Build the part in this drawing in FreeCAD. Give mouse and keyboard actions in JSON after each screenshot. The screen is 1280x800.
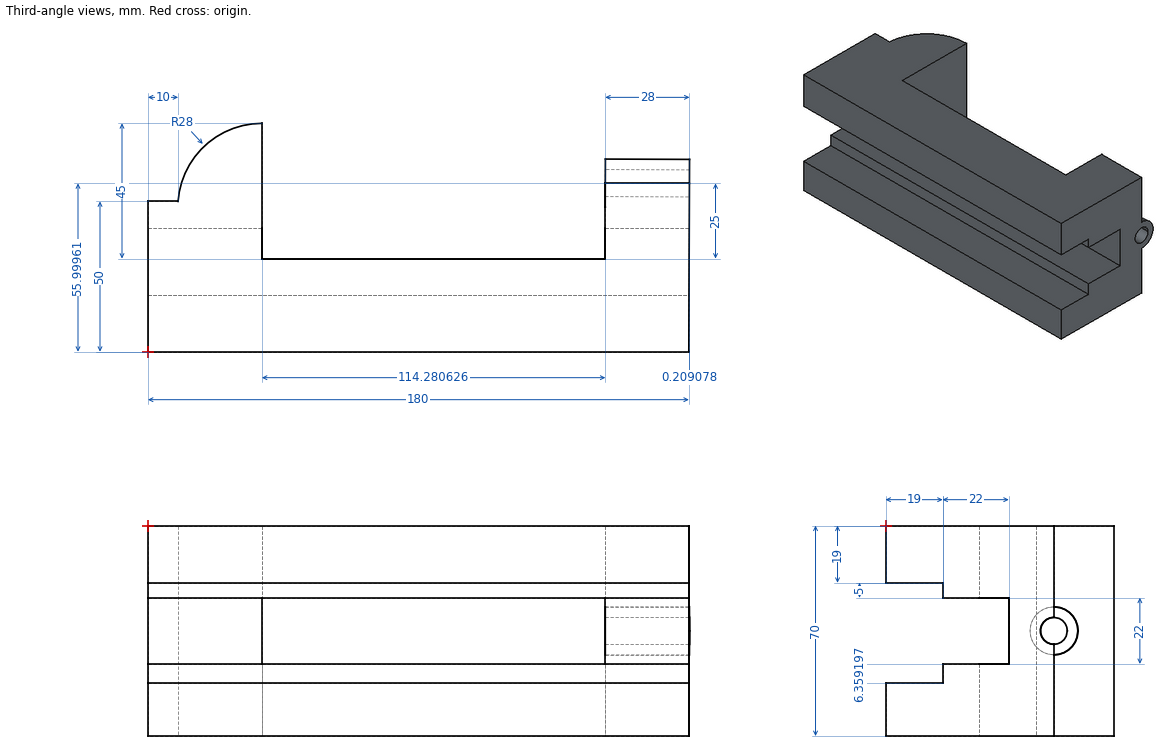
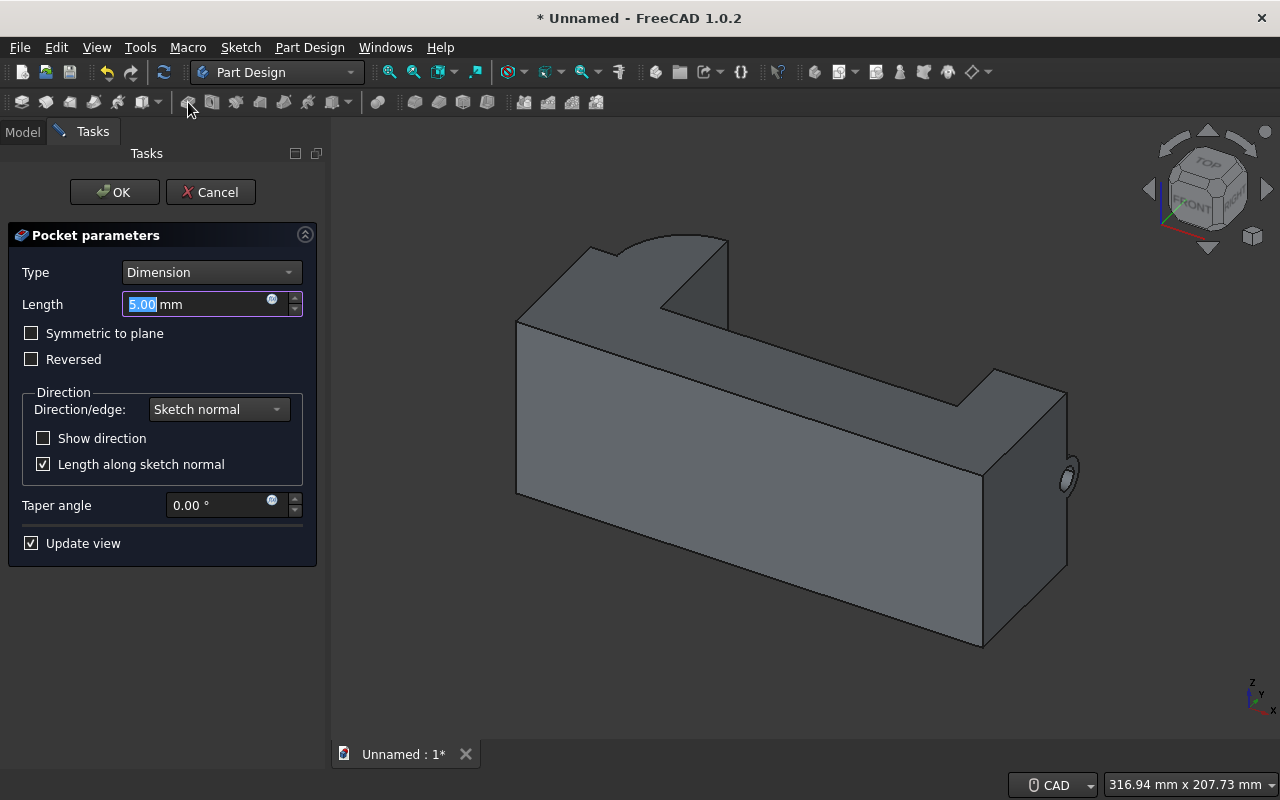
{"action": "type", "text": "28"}
{"action": "key", "text": "Tab"}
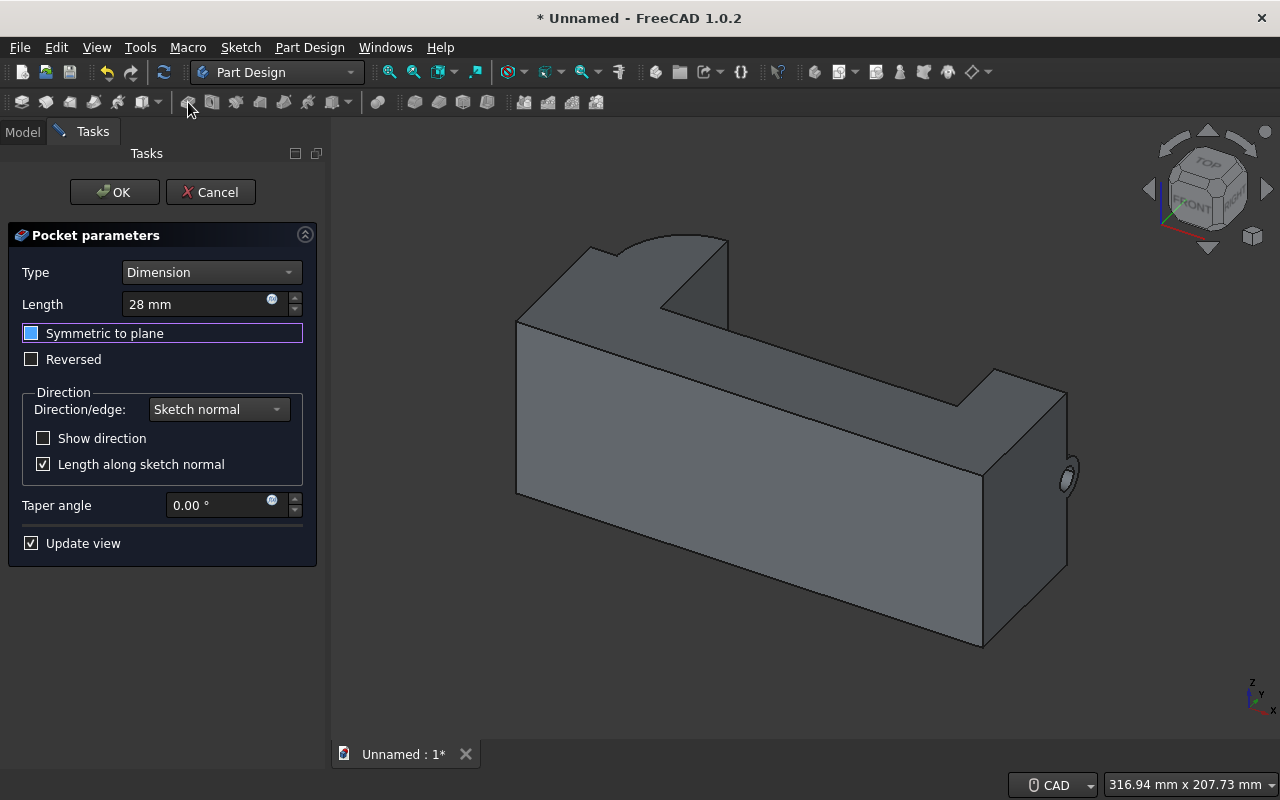
{"action": "left_click", "coordinate": [115, 192]}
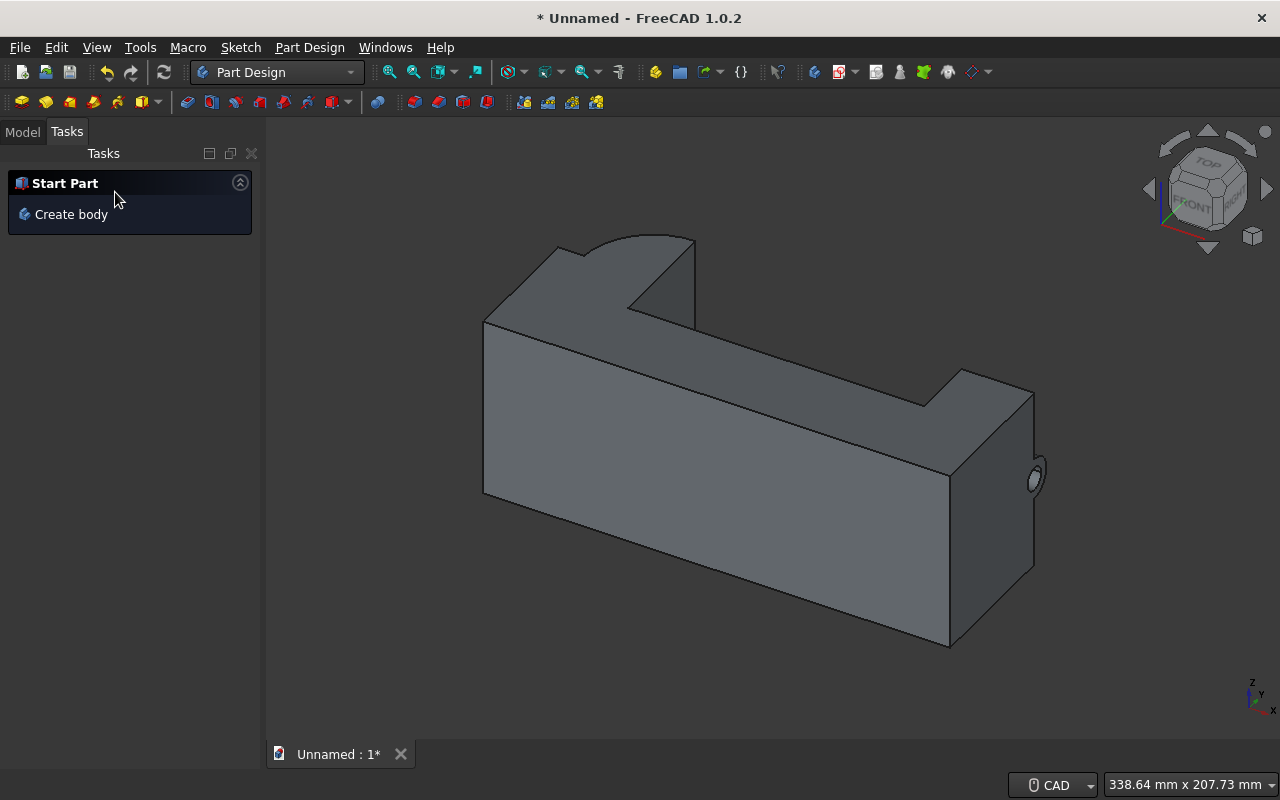
{"action": "left_click", "coordinate": [840, 72]}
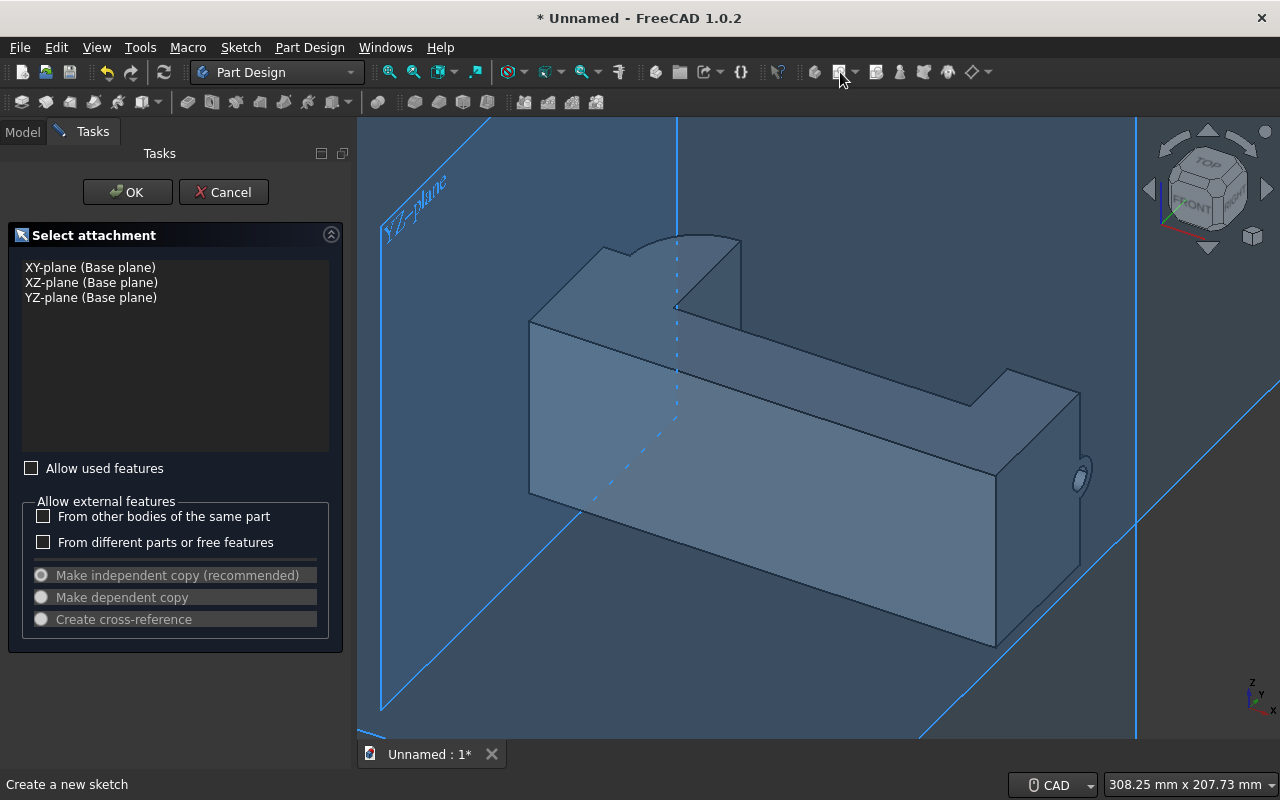
{"action": "left_click", "coordinate": [82, 298]}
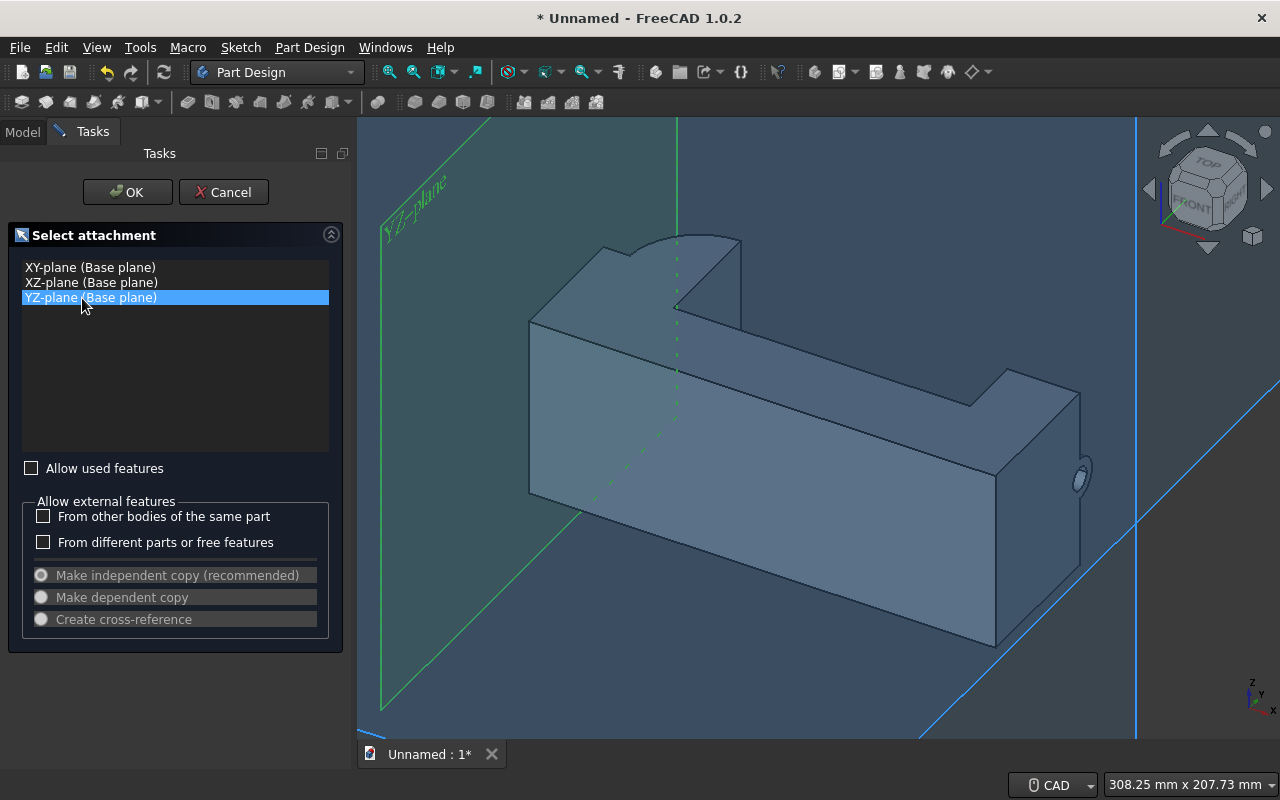
{"action": "left_click", "coordinate": [128, 192]}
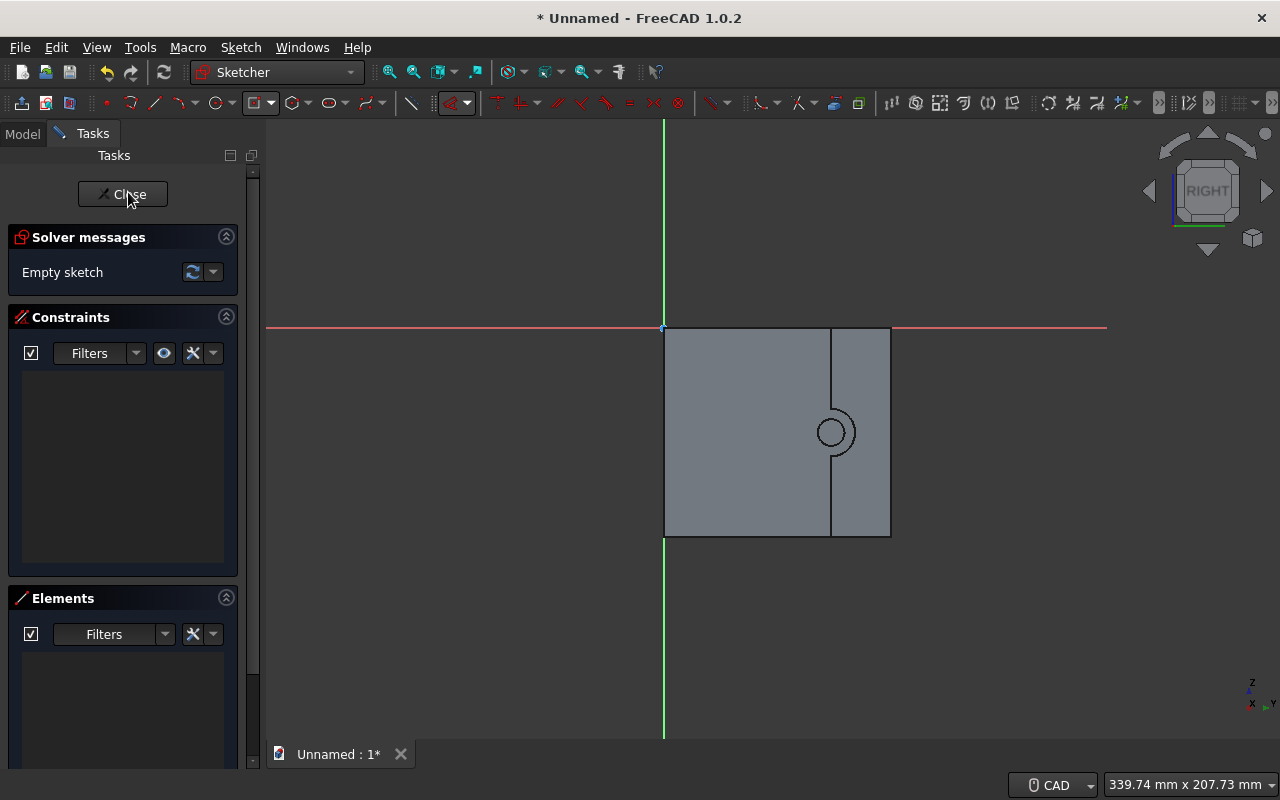
{"action": "left_click", "coordinate": [70, 104]}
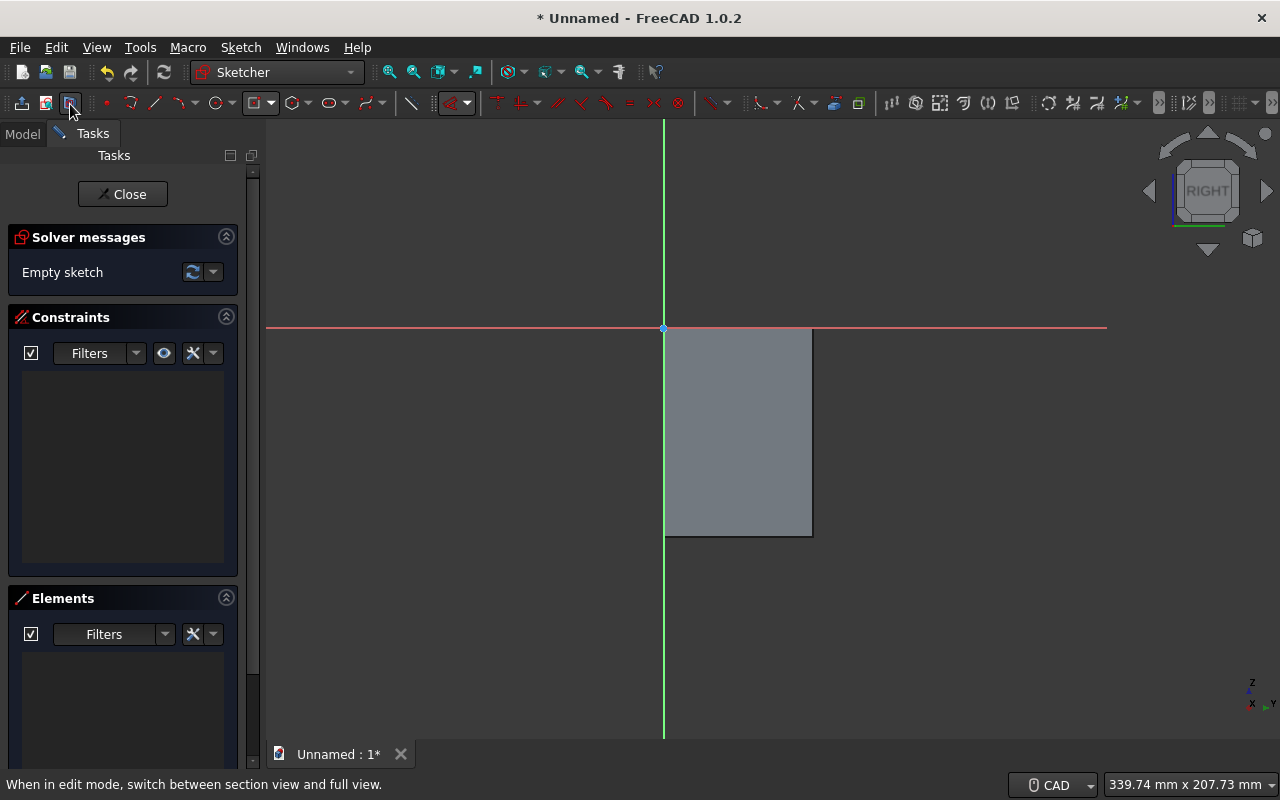
{"action": "scroll", "coordinate": [737, 393], "scroll_direction": "up", "scroll_amount": 5}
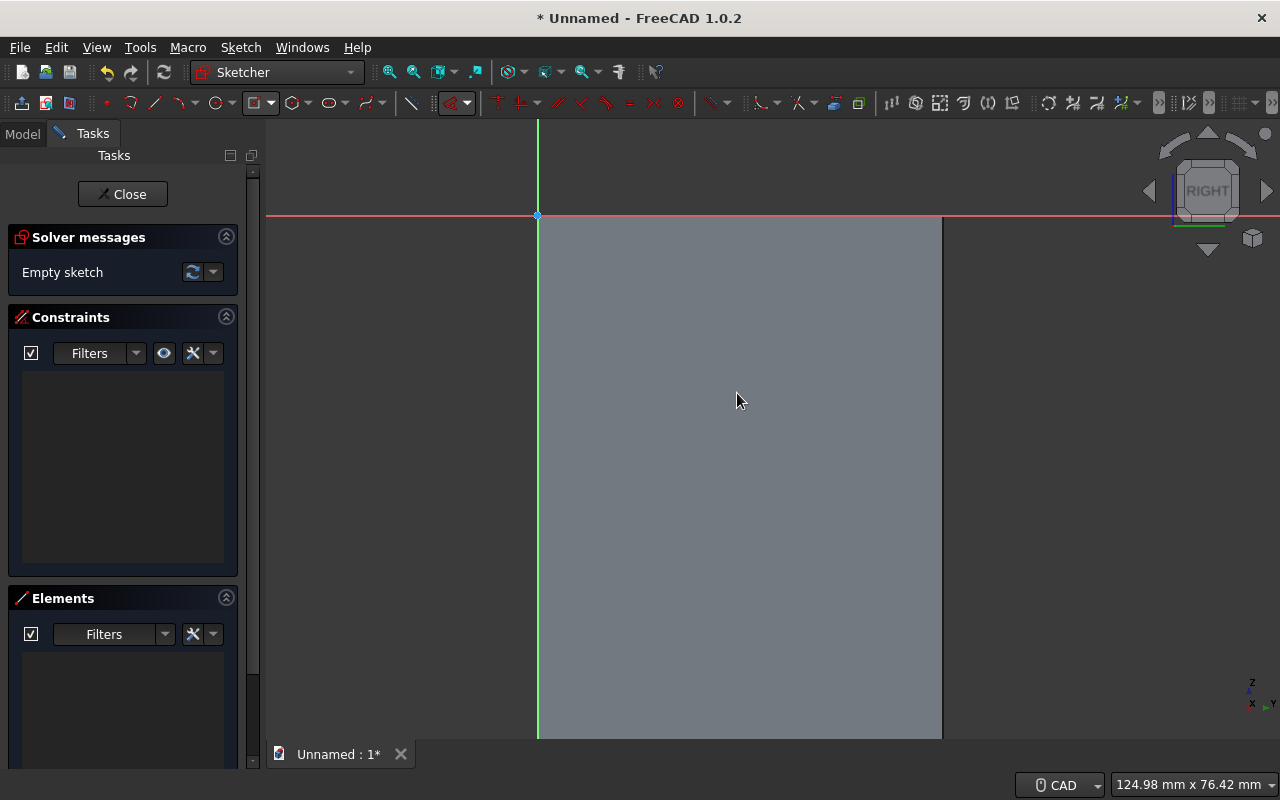
{"action": "left_click", "coordinate": [132, 104]}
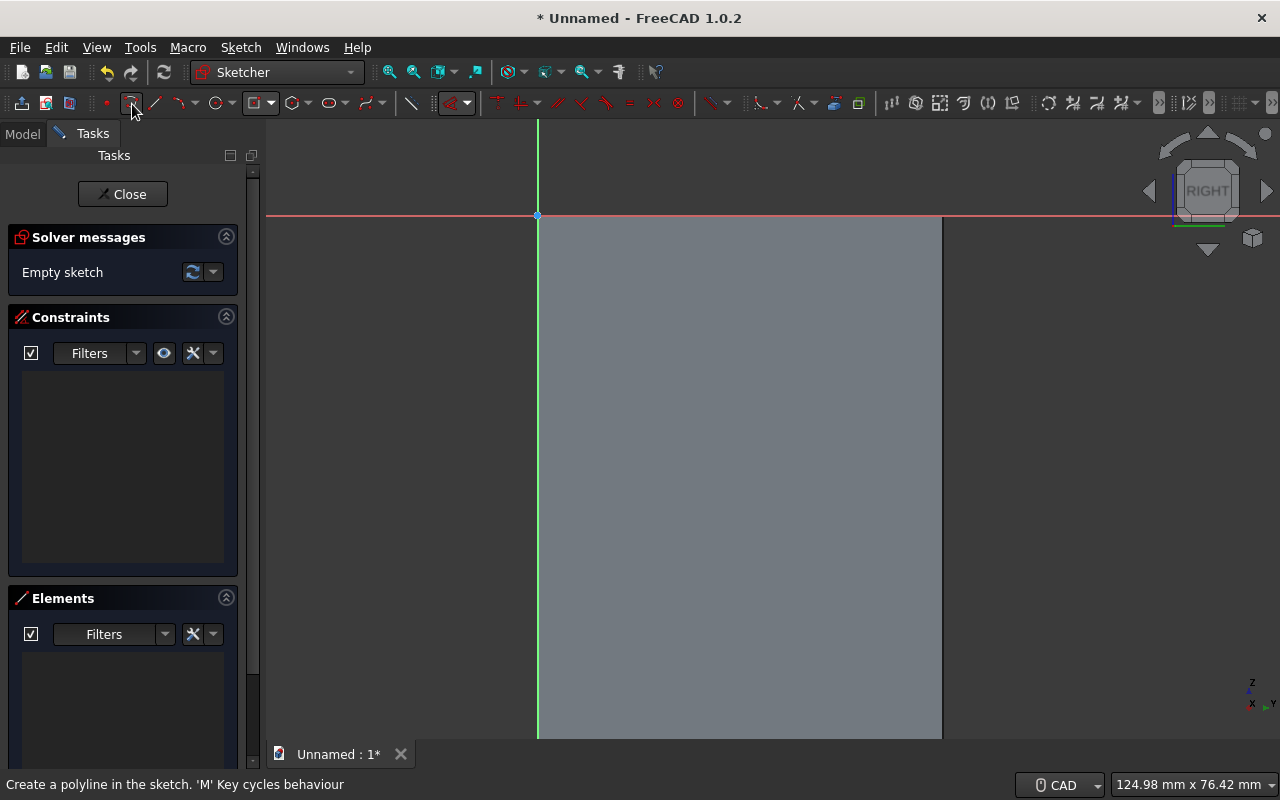
{"action": "left_click", "coordinate": [538, 370]}
{"action": "left_click", "coordinate": [692, 370]}
{"action": "left_click", "coordinate": [692, 410]}
{"action": "left_click", "coordinate": [870, 410]}
{"action": "left_click", "coordinate": [870, 589]}
{"action": "left_click", "coordinate": [692, 589]}
{"action": "left_click", "coordinate": [692, 641]}
{"action": "left_click", "coordinate": [547, 641]}
{"action": "left_click", "coordinate": [538, 371]}
{"action": "key", "text": "Escape"}
{"action": "key", "text": "Escape"}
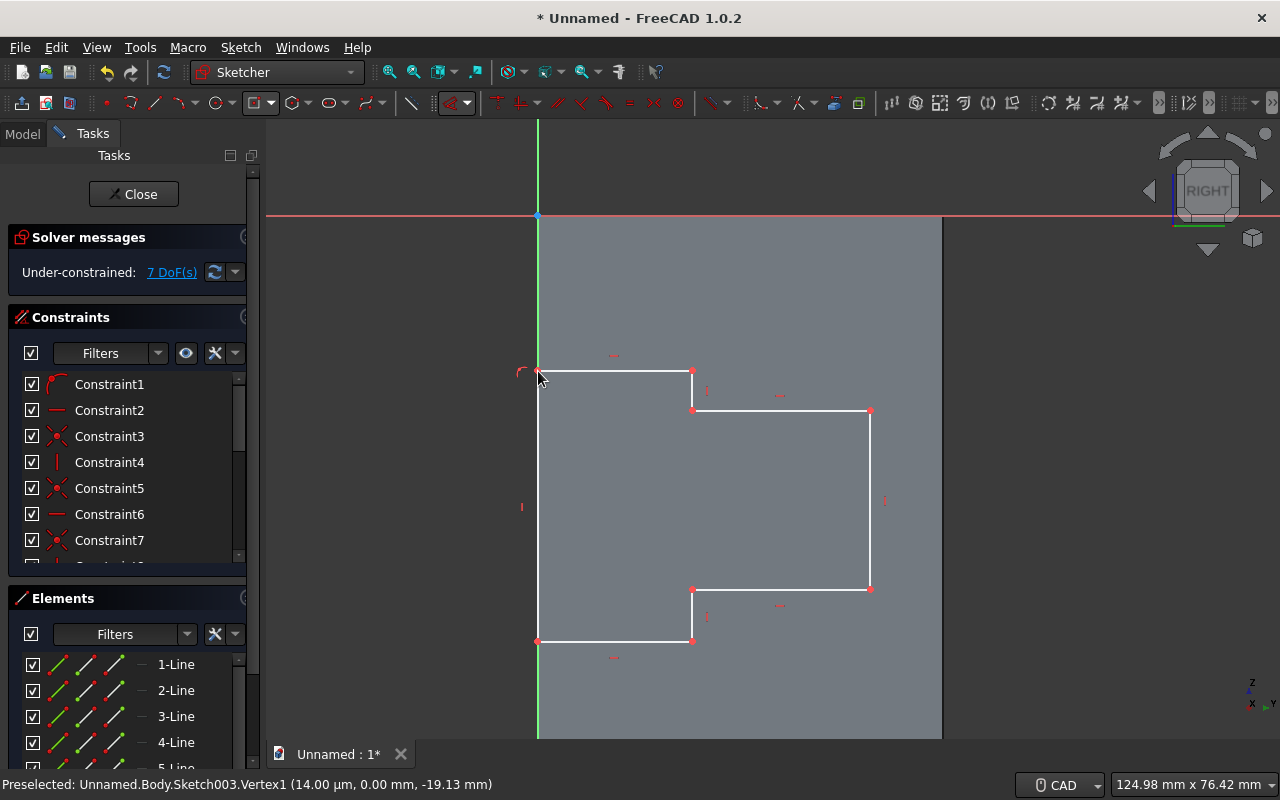
{"action": "left_click", "coordinate": [692, 383]}